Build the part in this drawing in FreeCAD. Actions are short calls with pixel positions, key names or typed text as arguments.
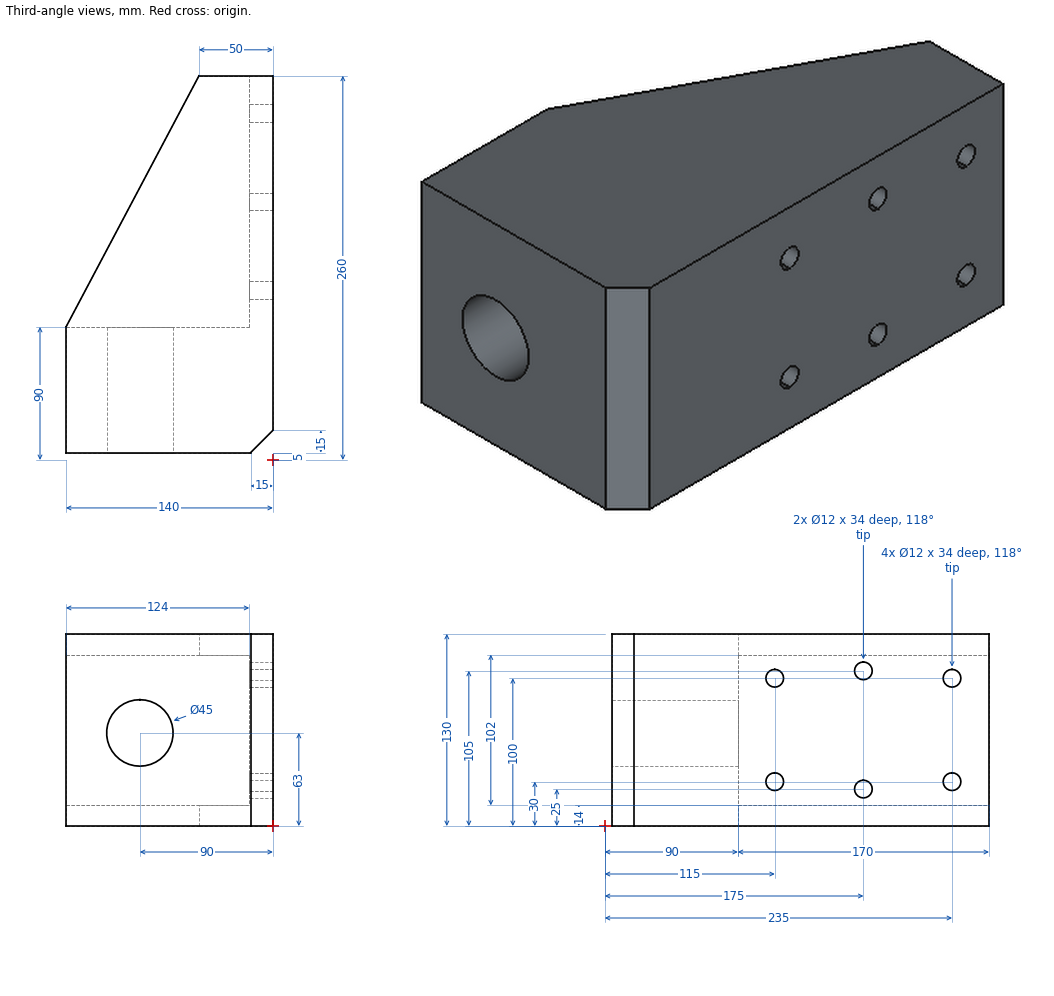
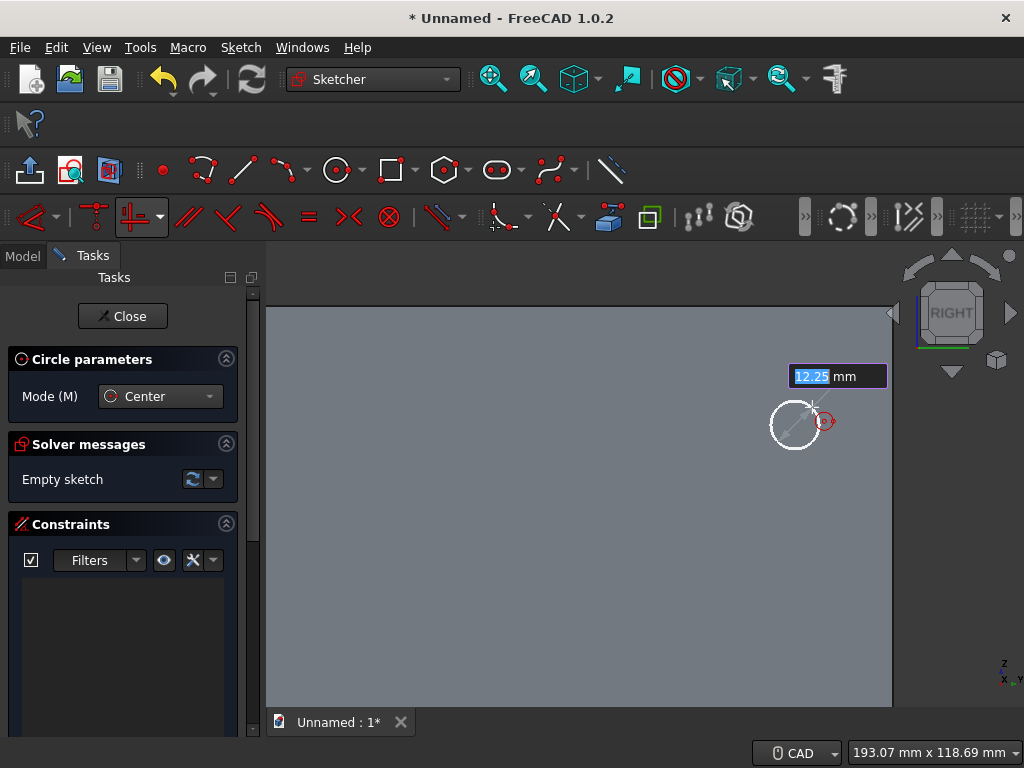
text(12)
key(Return)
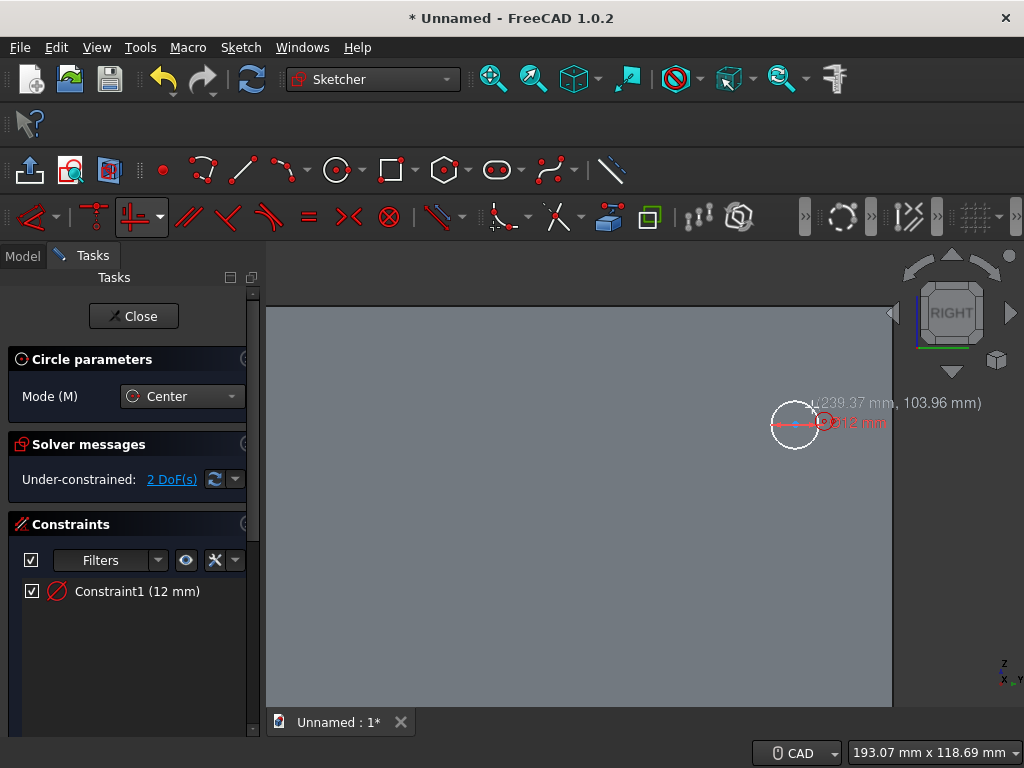
scroll(765, 365, down, 4)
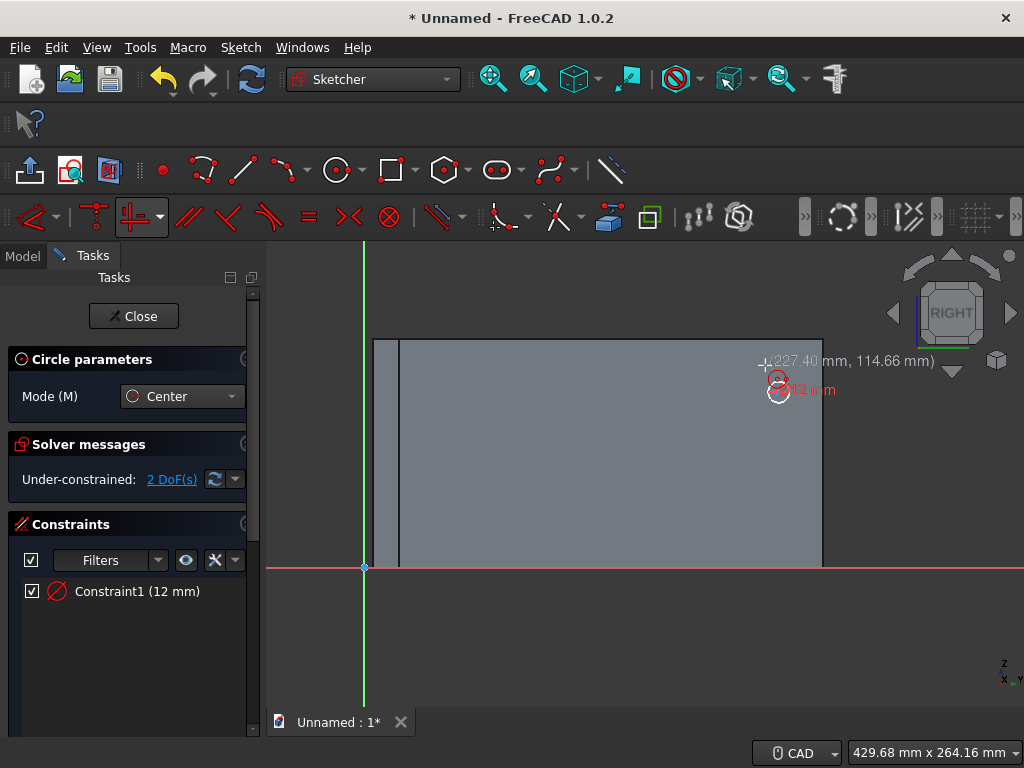
scroll(779, 515, up, 4)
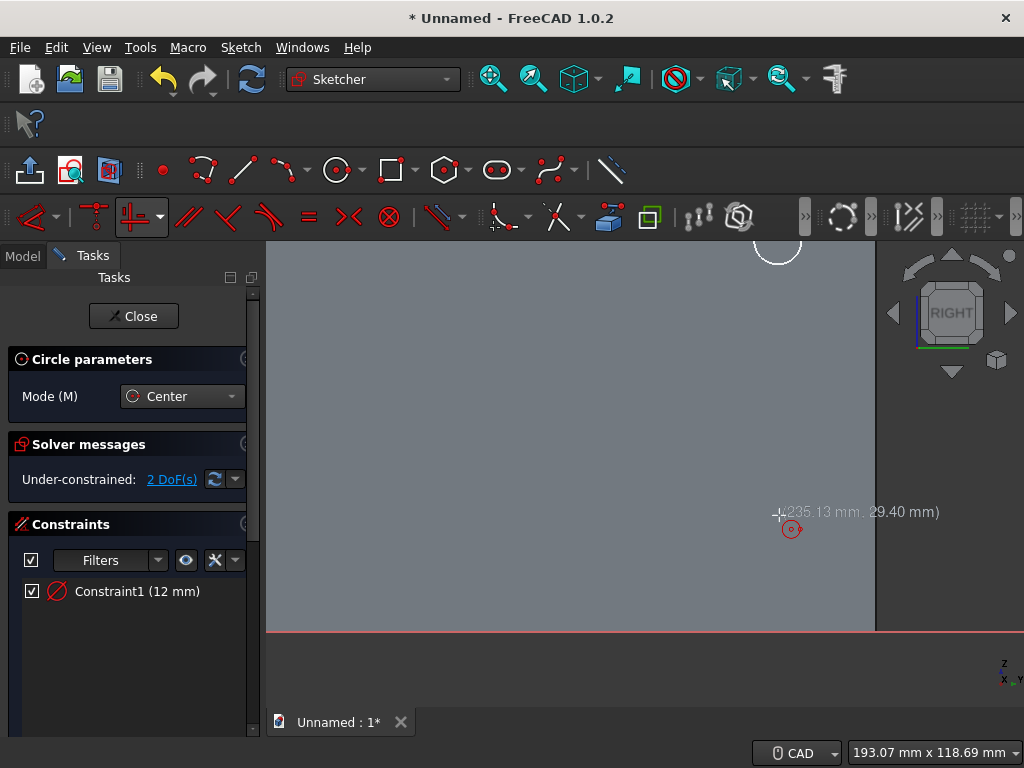
click(778, 514)
move(794, 497)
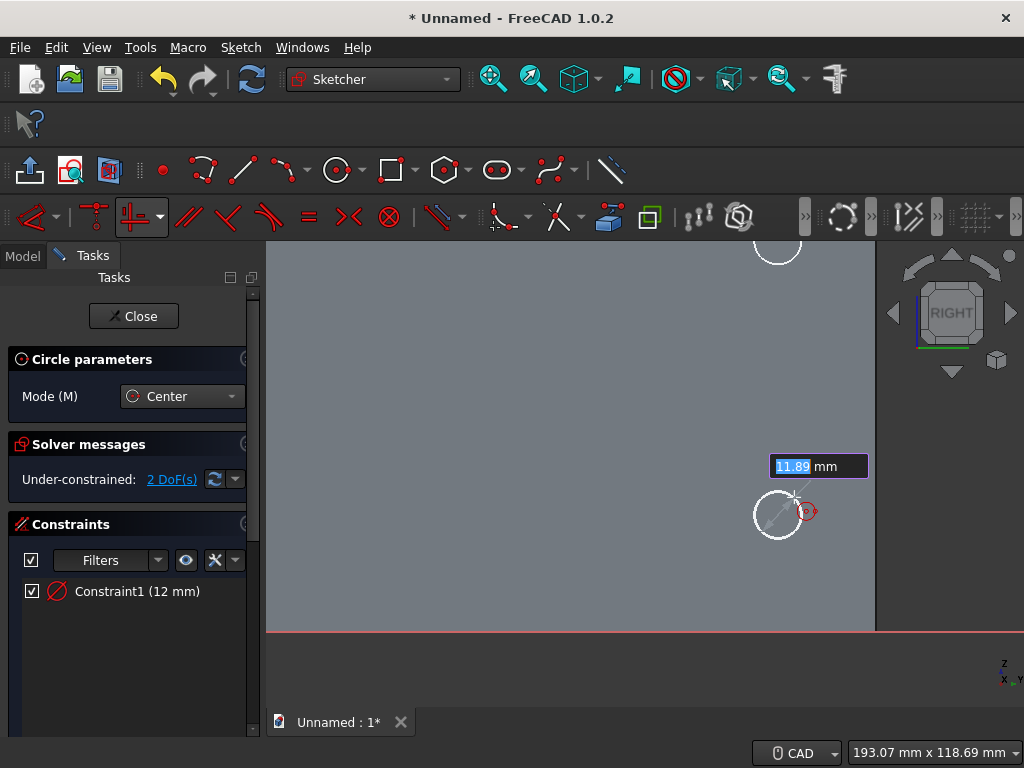
text(12)
key(Return)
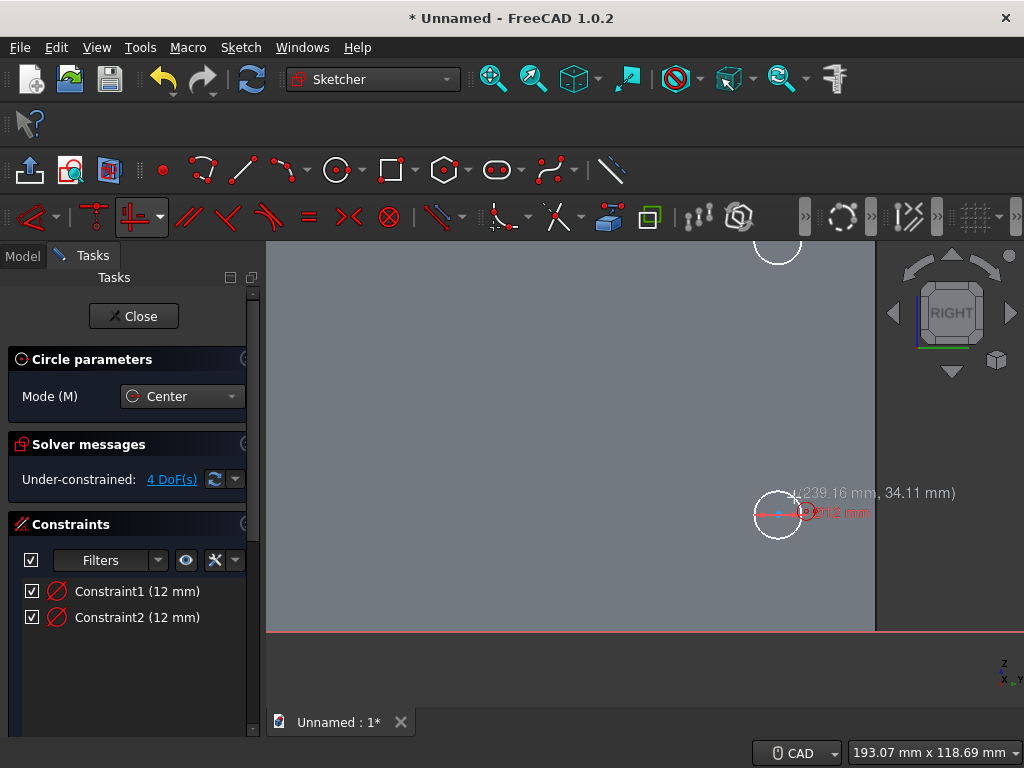
scroll(779, 515, down, 4)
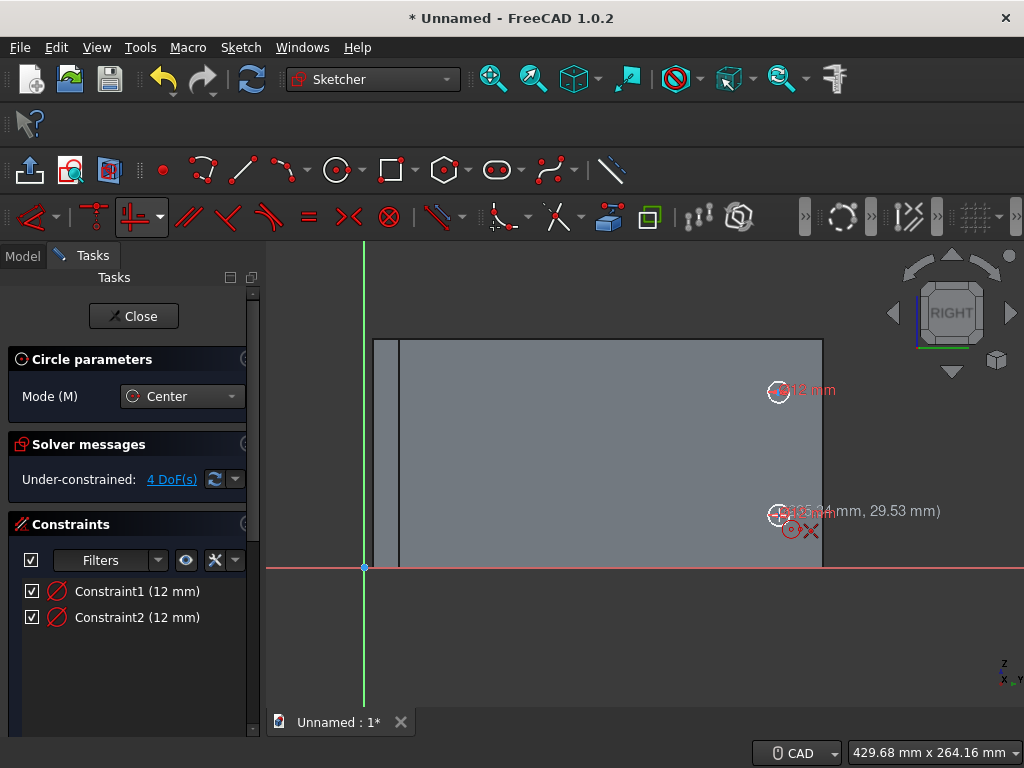
scroll(567, 391, up, 4)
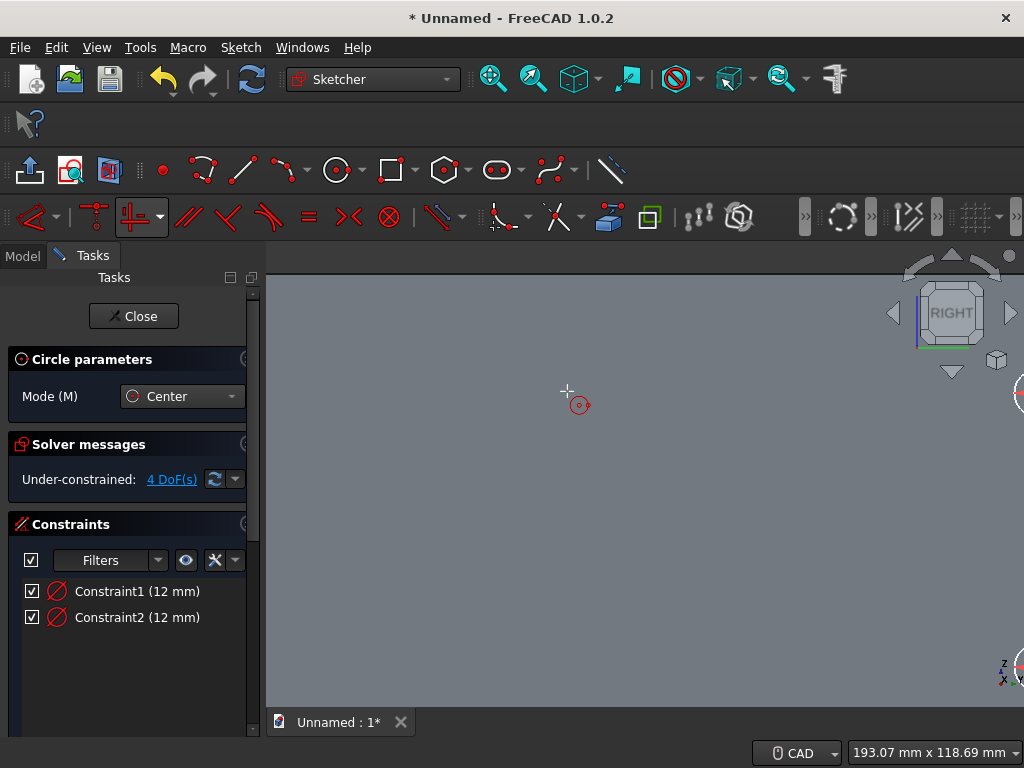
click(567, 392)
move(583, 375)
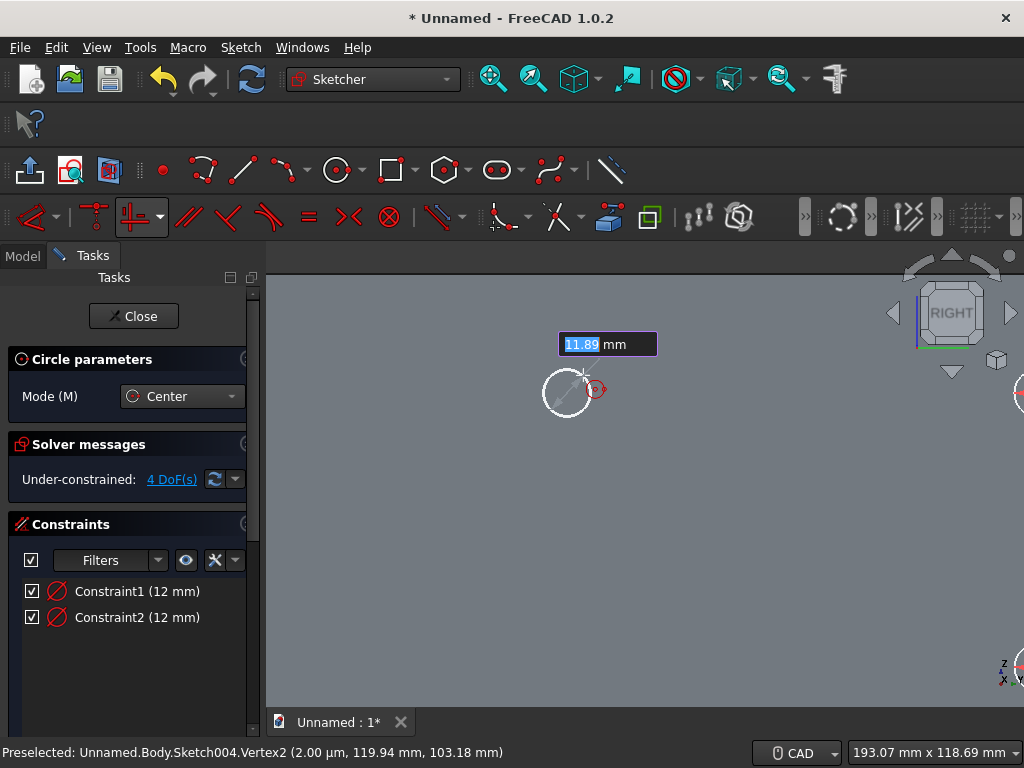
text(12)
key(Return)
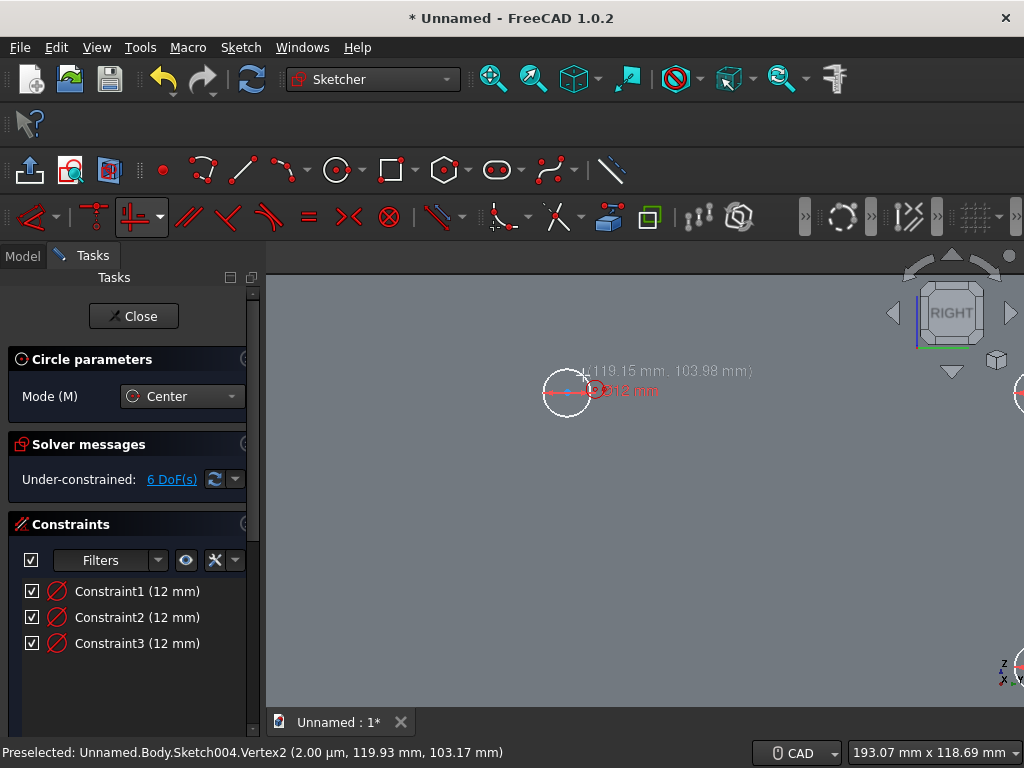
click(567, 666)
move(583, 650)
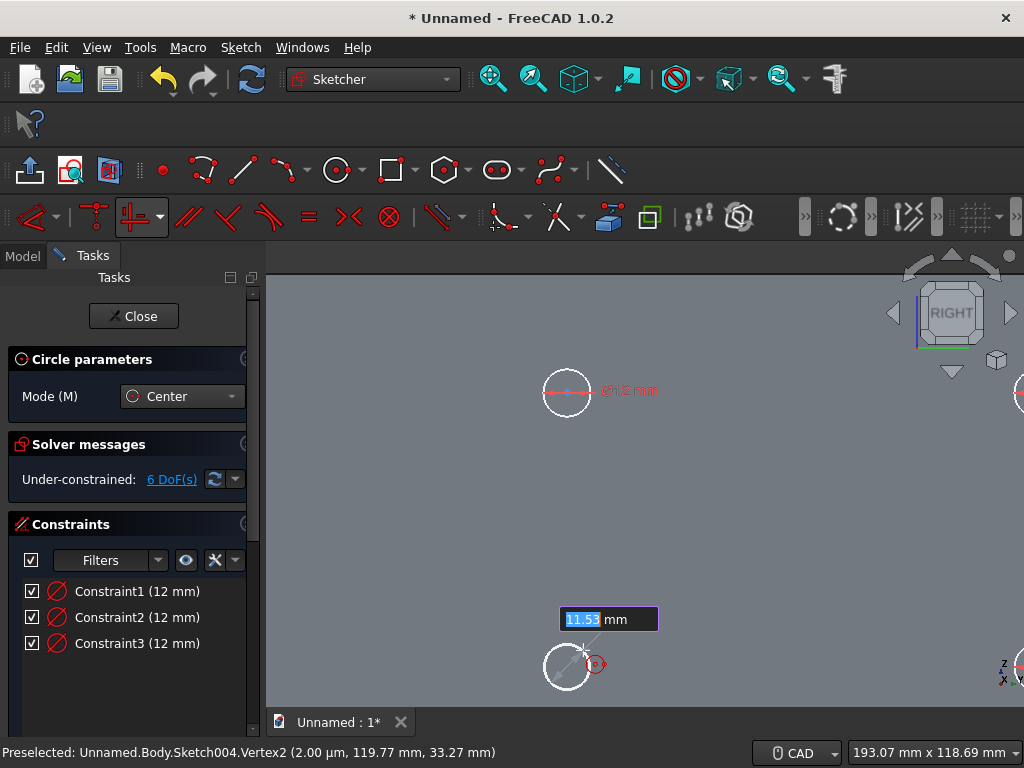
text(12)
key(Return)
key(Escape)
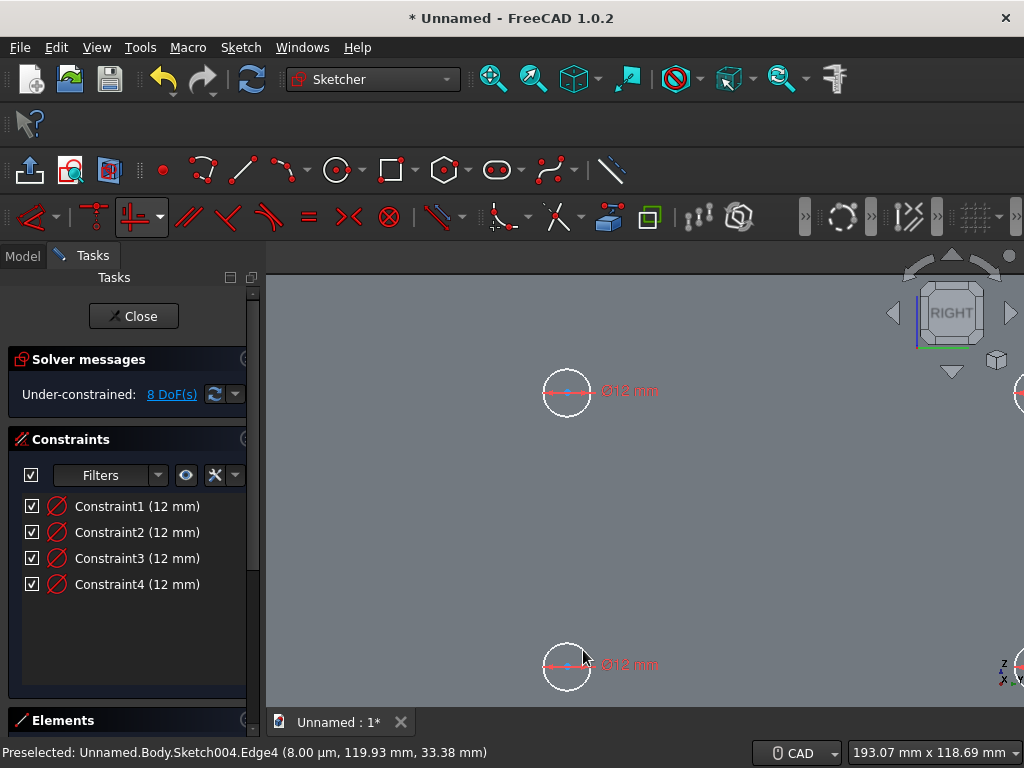
scroll(567, 391, down, 4)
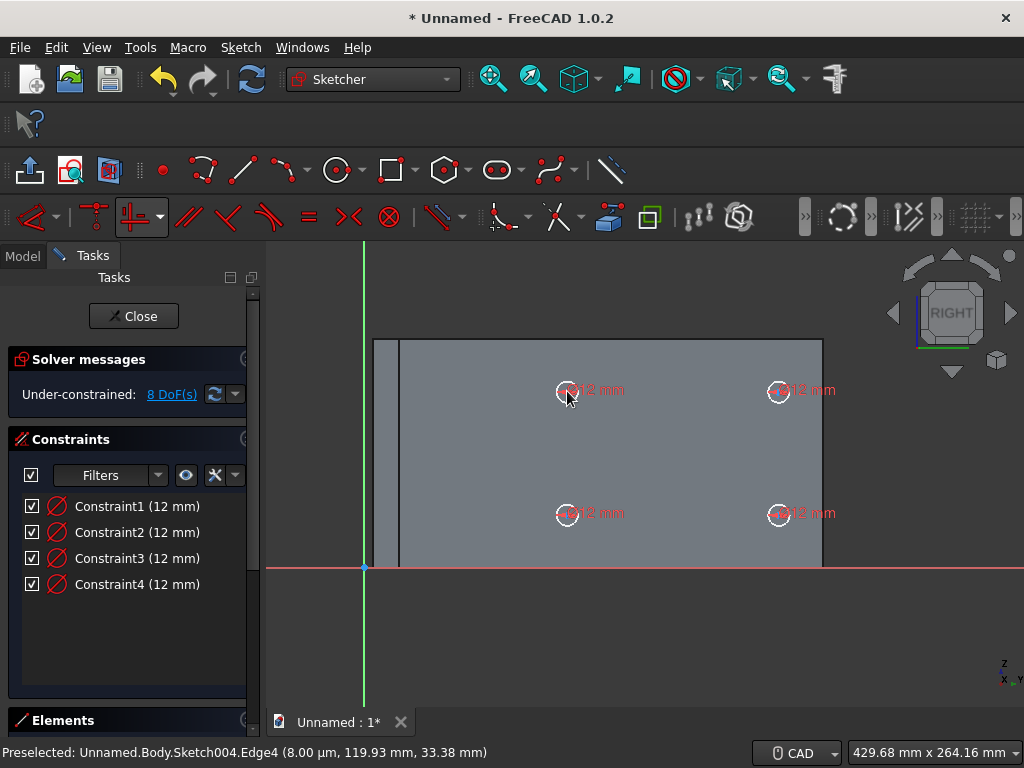
click(779, 392)